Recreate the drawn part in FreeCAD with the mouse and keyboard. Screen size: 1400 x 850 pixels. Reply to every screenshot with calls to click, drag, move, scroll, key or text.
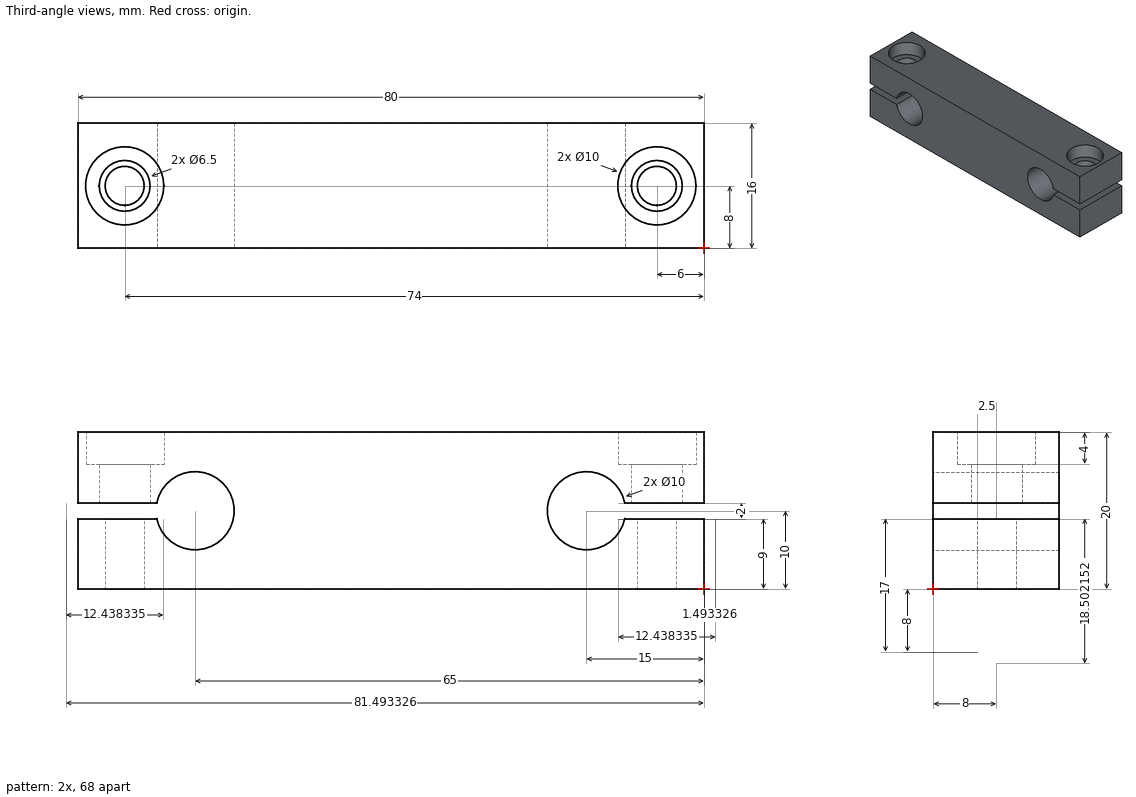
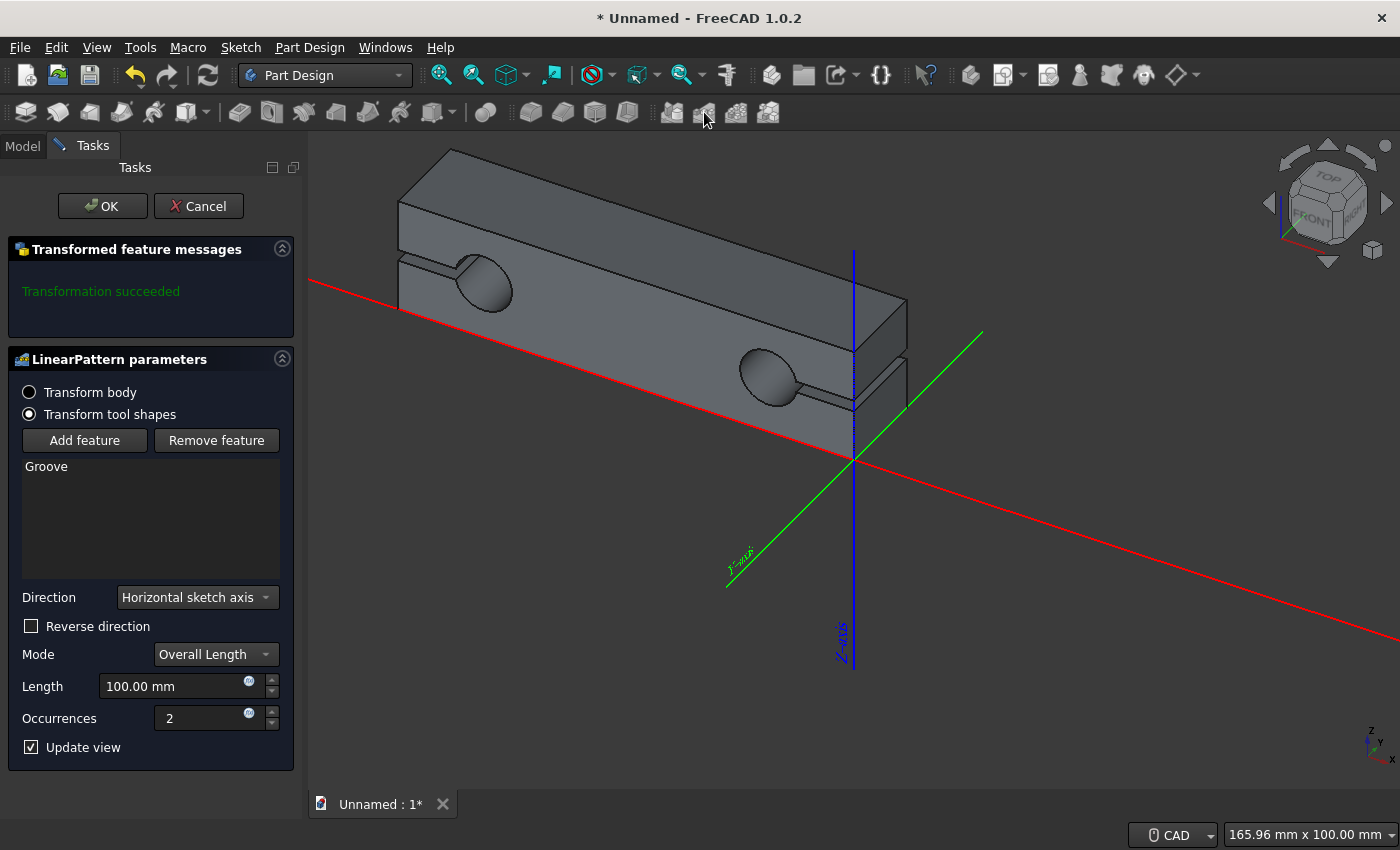
click(198, 598)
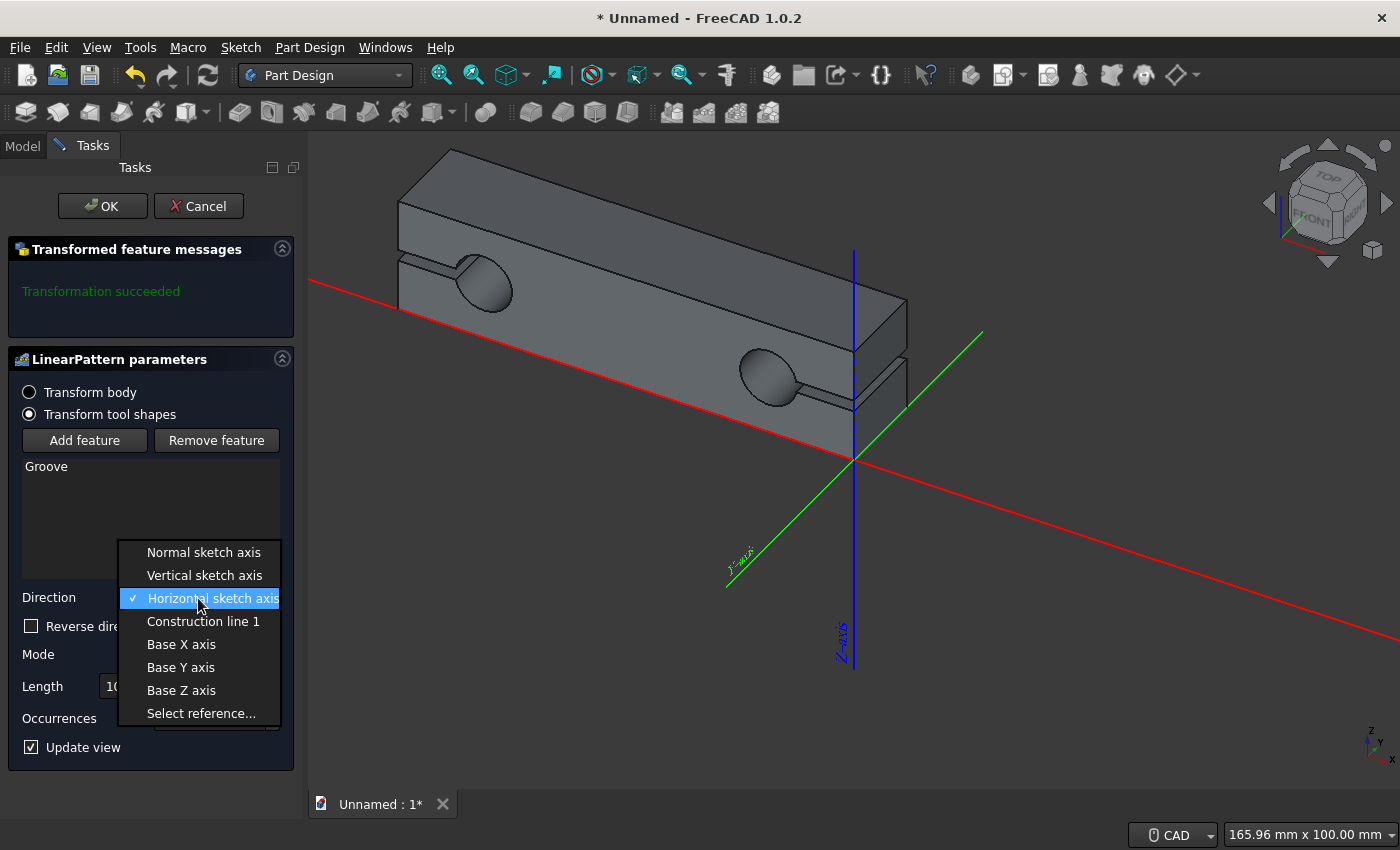
click(198, 644)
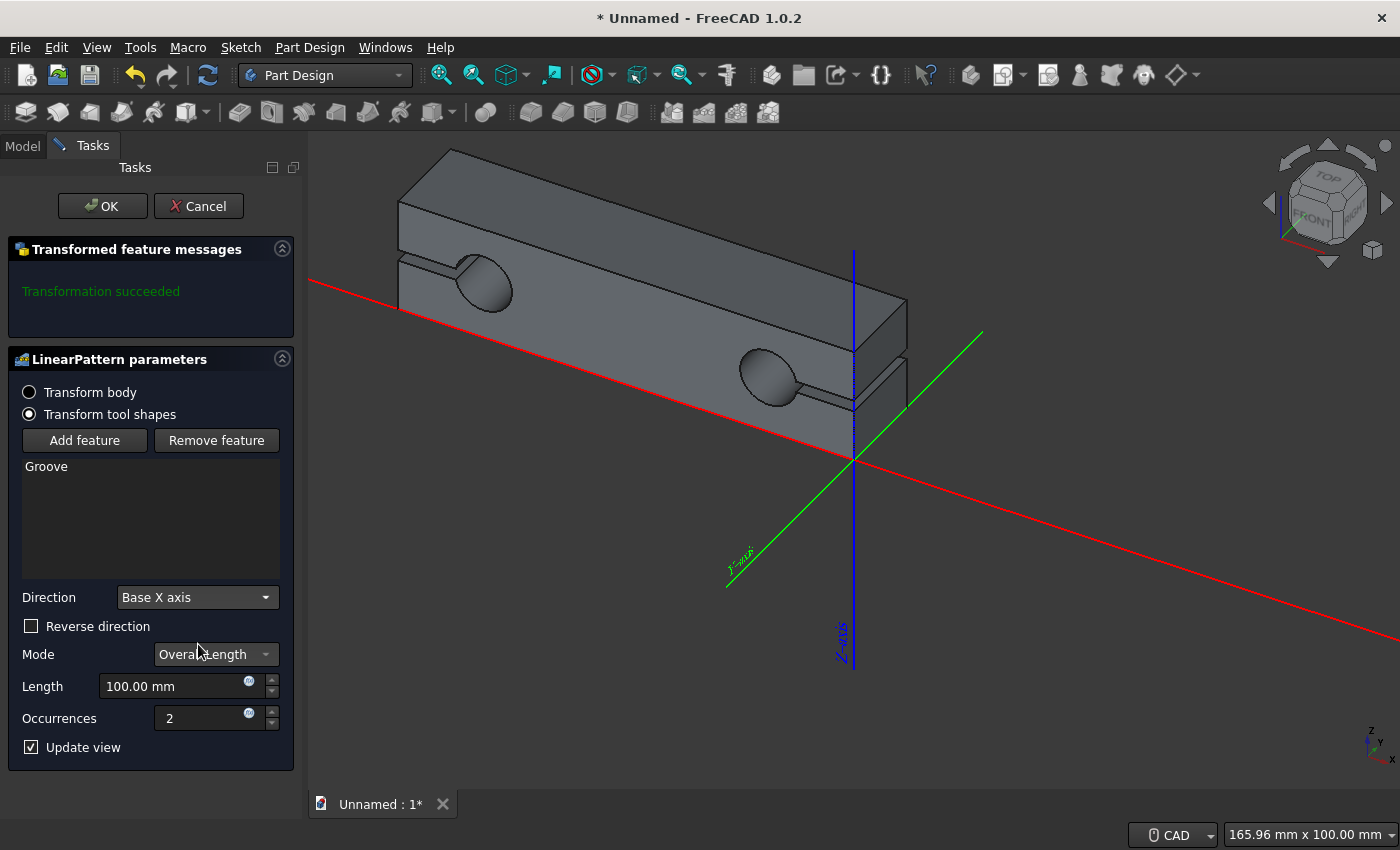
click(217, 654)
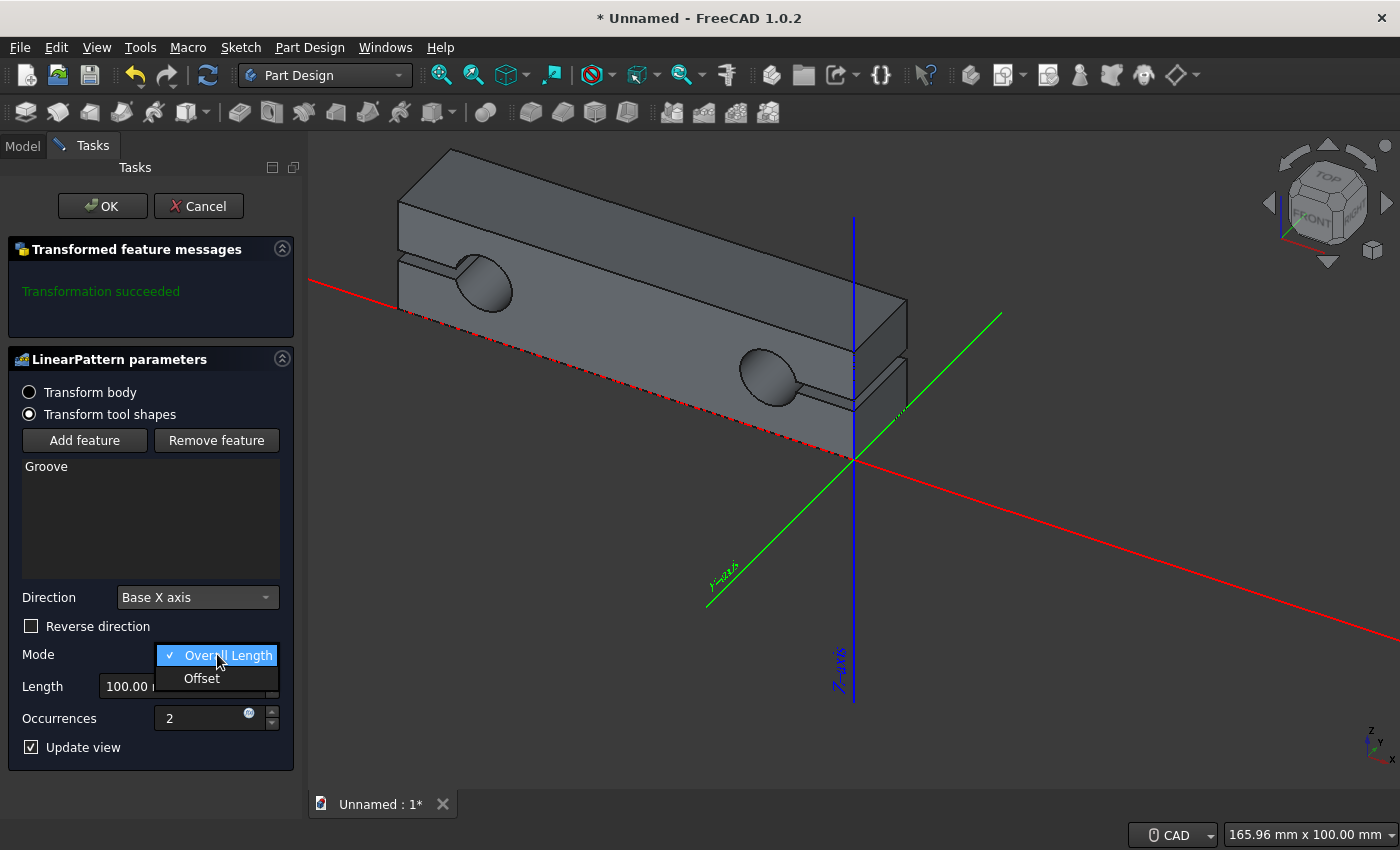
click(216, 678)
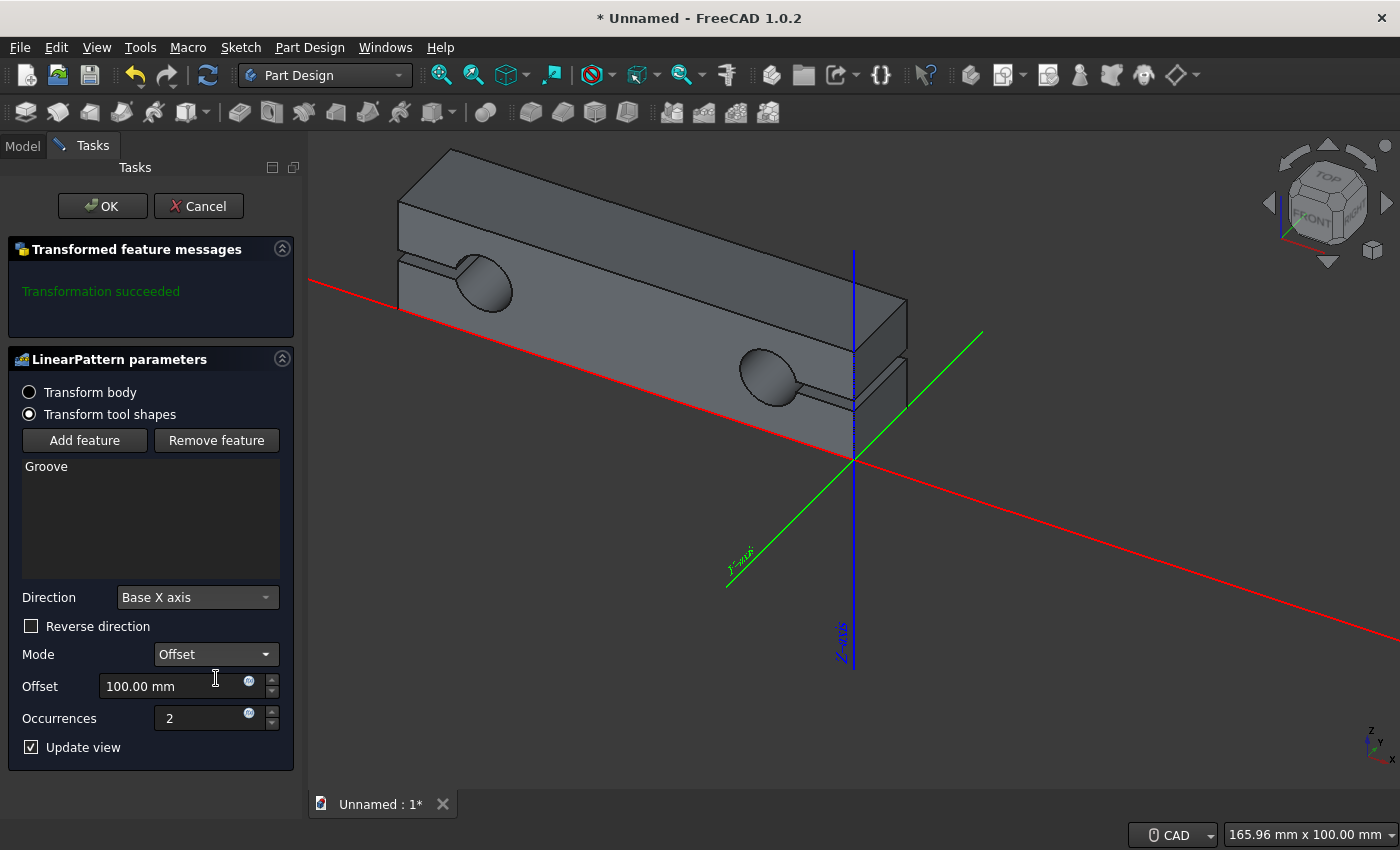
triple_click(182, 686)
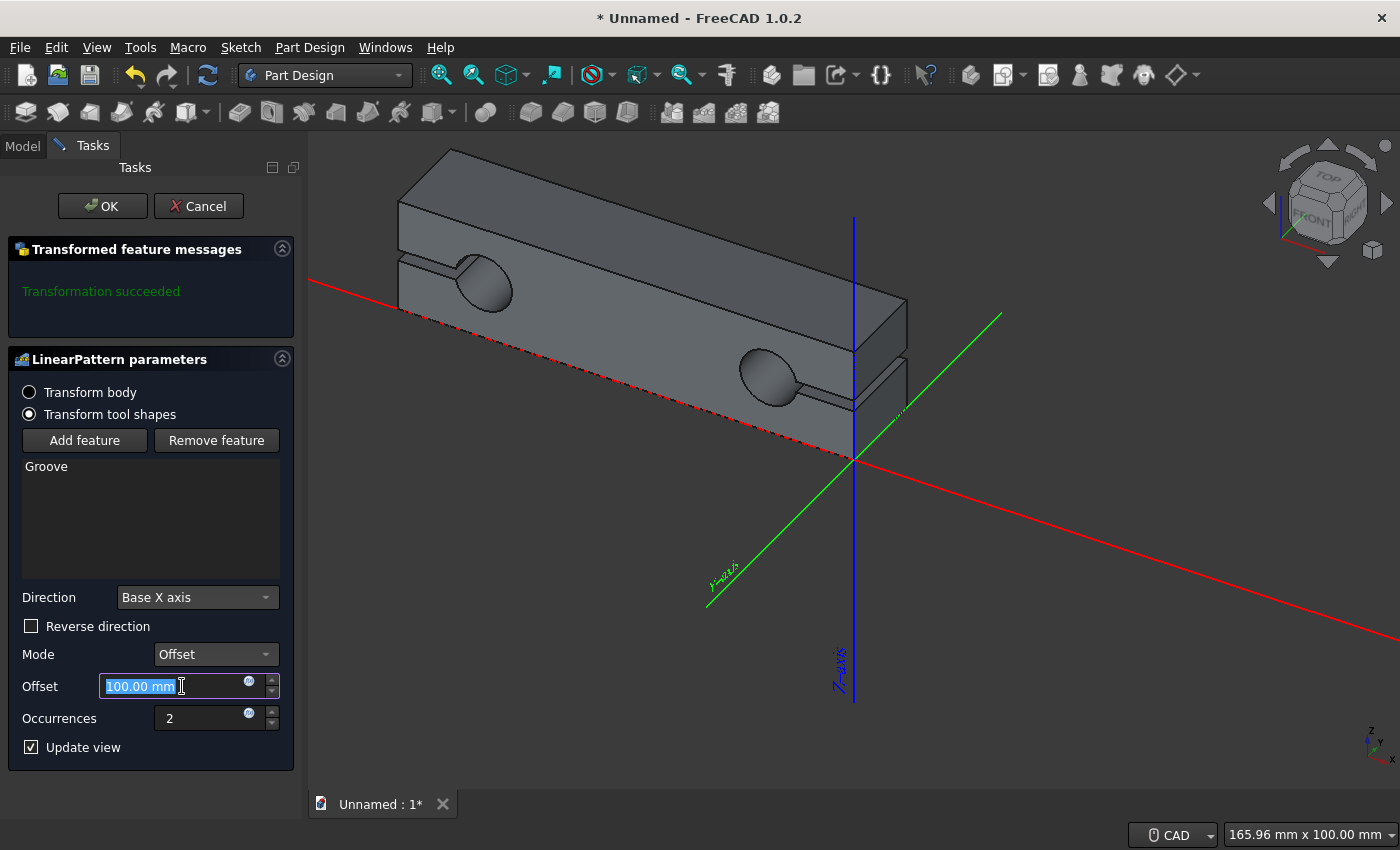
text(68)
key(Tab)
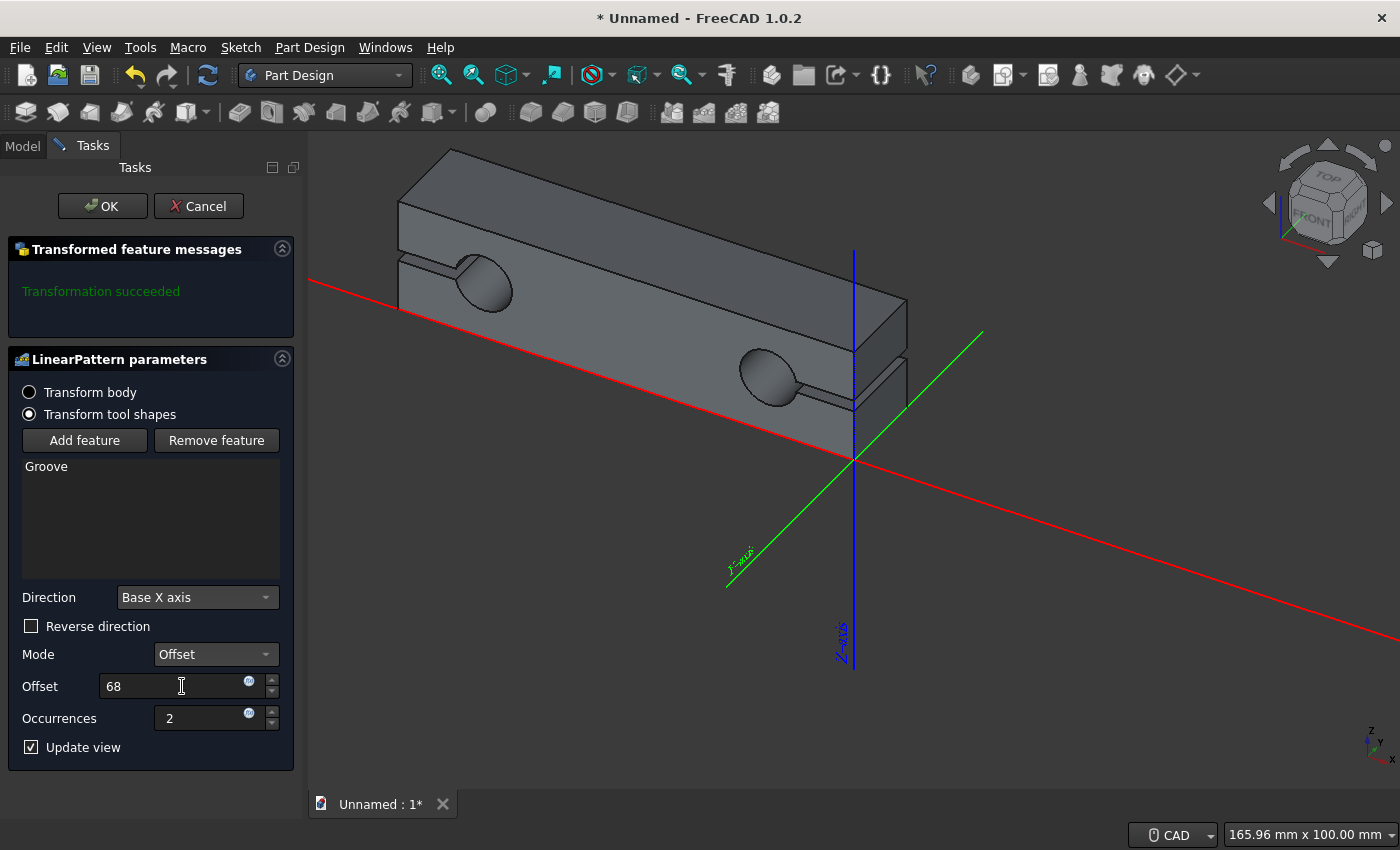
triple_click(209, 718)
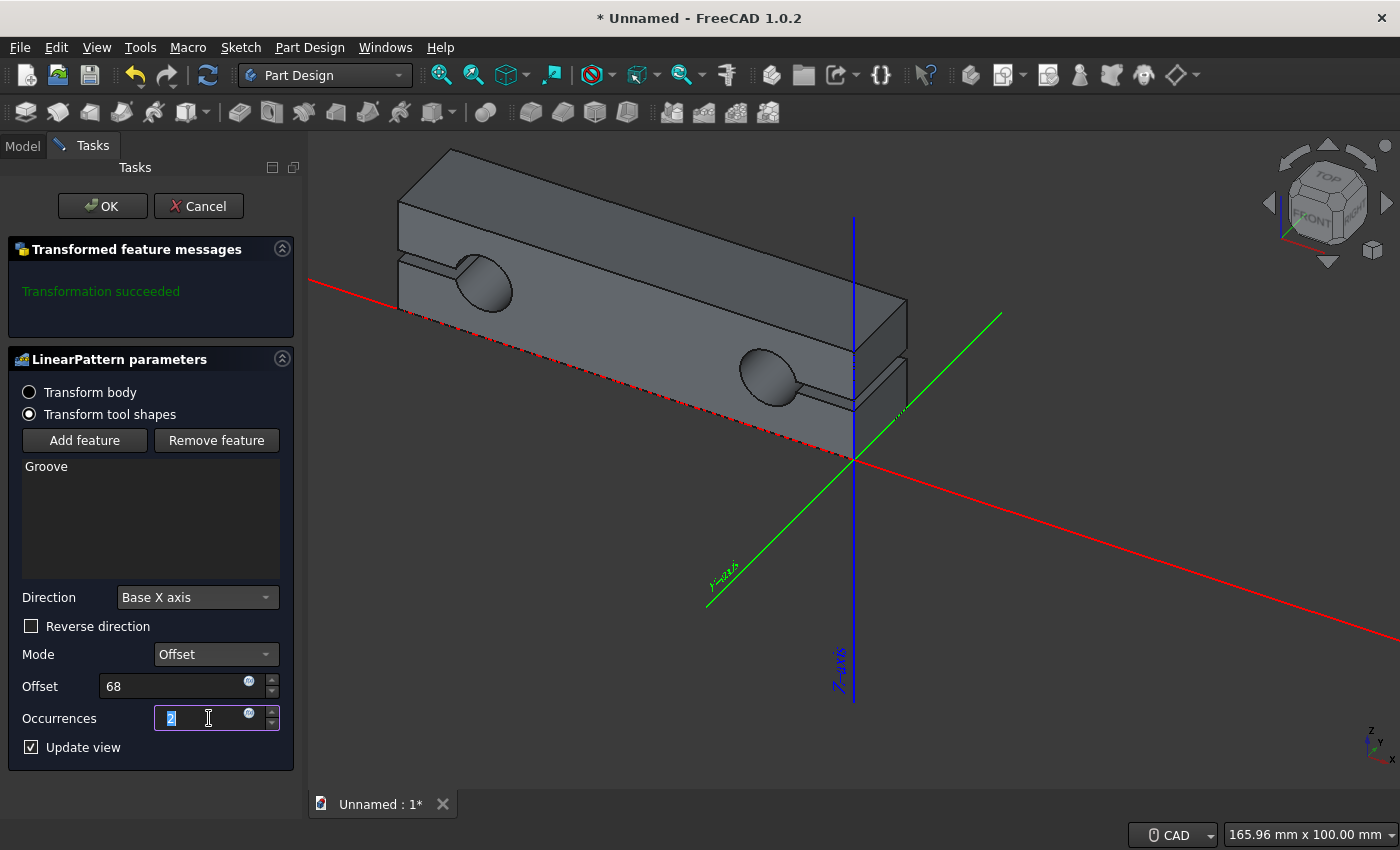
text(2)
key(Tab)